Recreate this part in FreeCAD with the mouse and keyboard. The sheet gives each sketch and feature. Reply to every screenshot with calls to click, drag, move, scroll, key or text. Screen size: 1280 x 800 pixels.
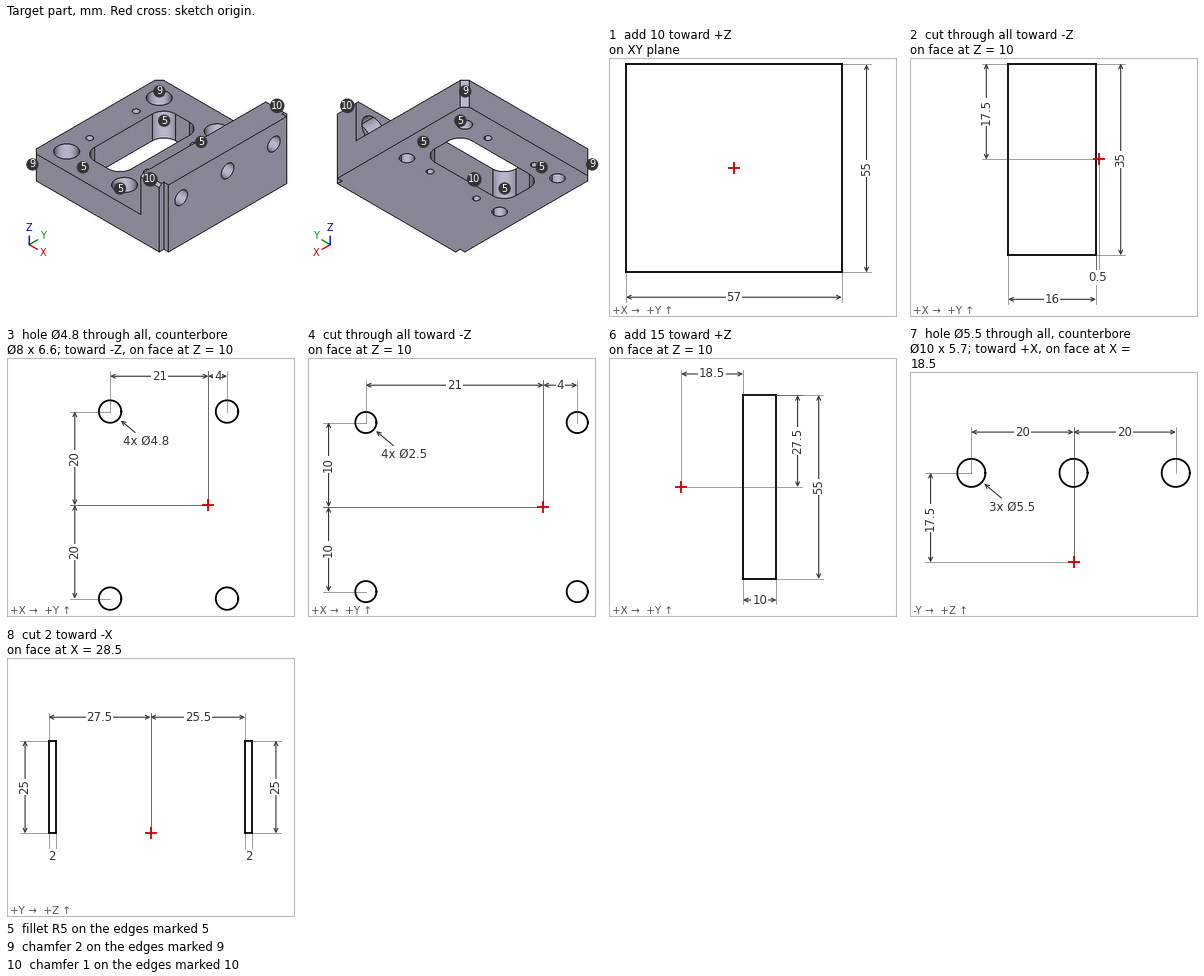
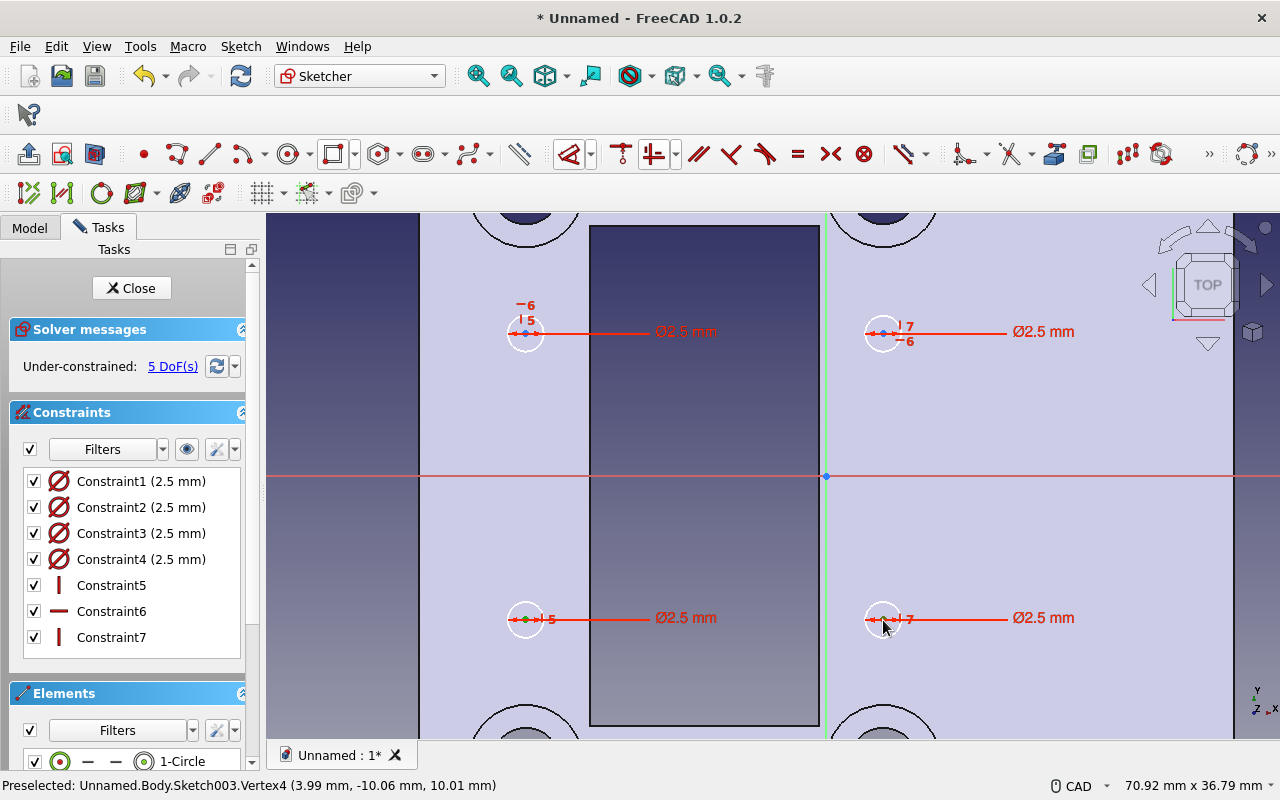
click(676, 154)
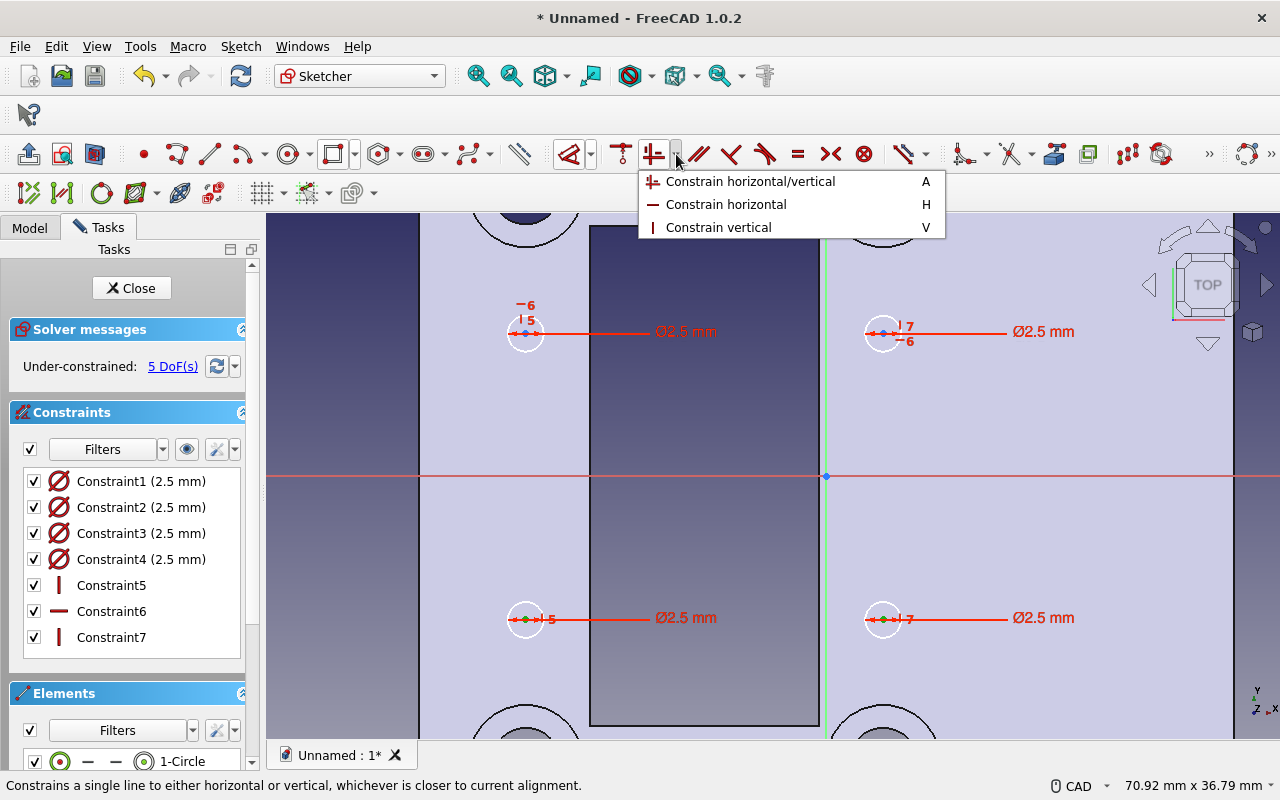
click(792, 204)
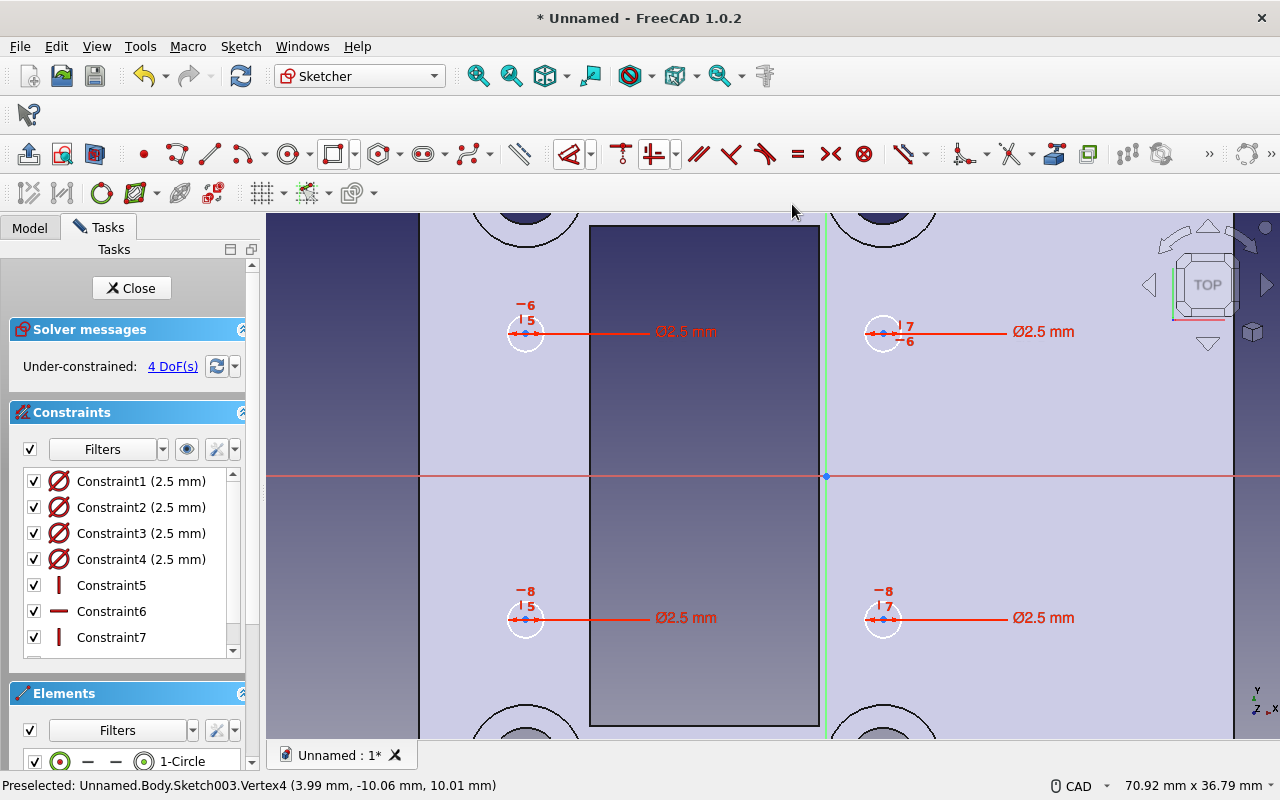
click(883, 334)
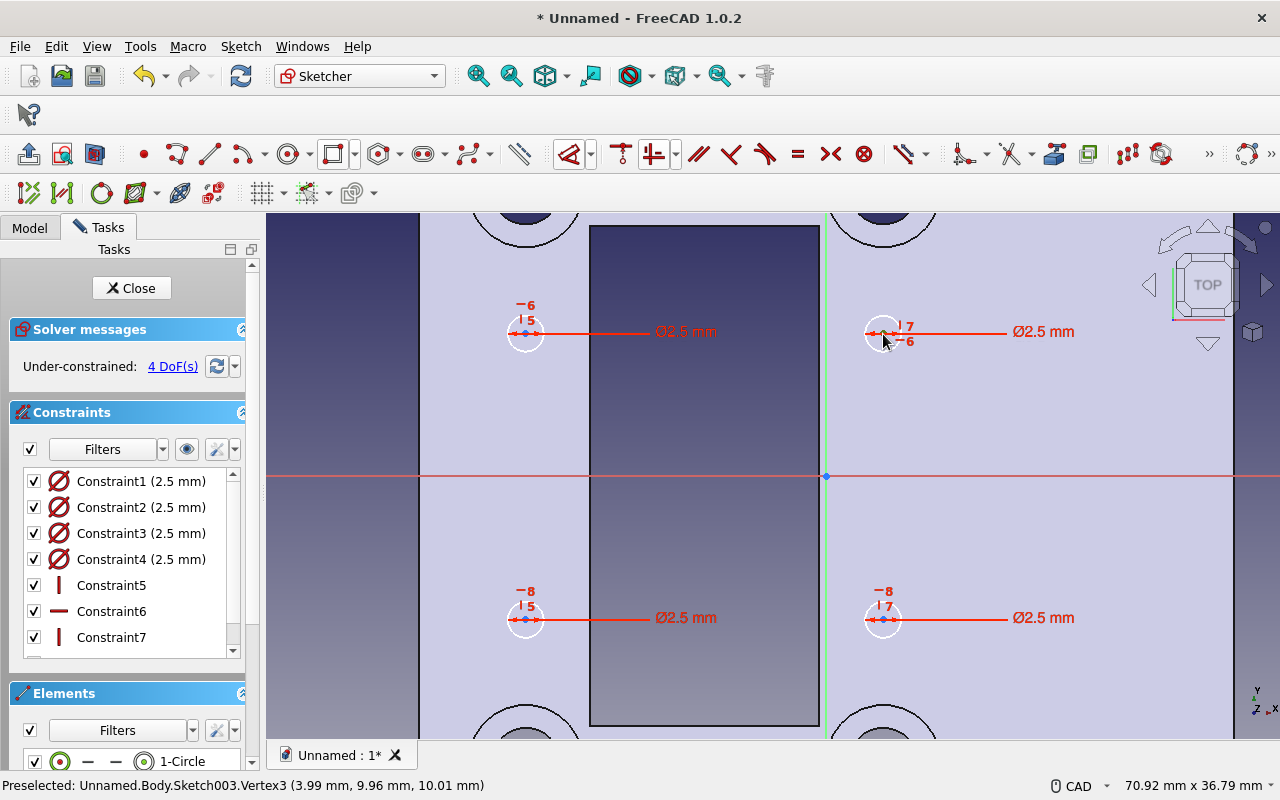
click(590, 154)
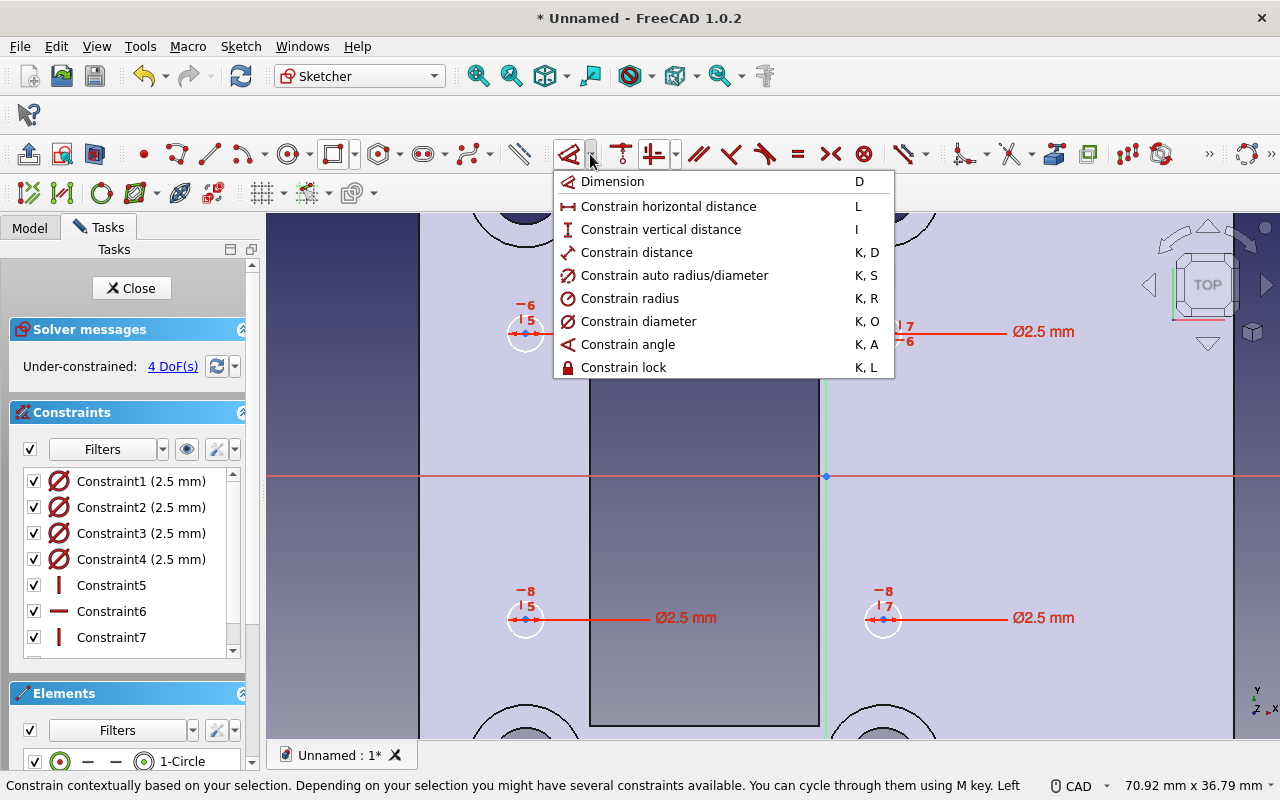
click(724, 206)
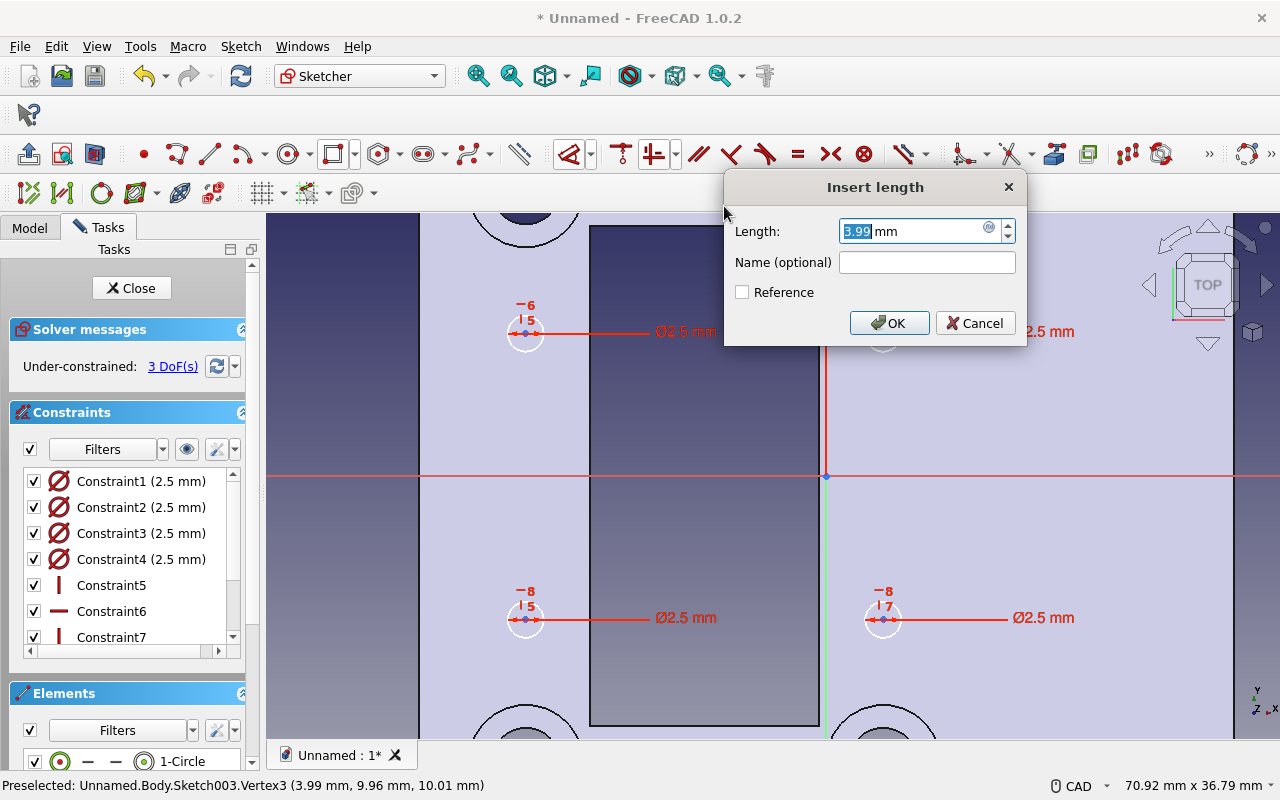
text(4)
key(Return)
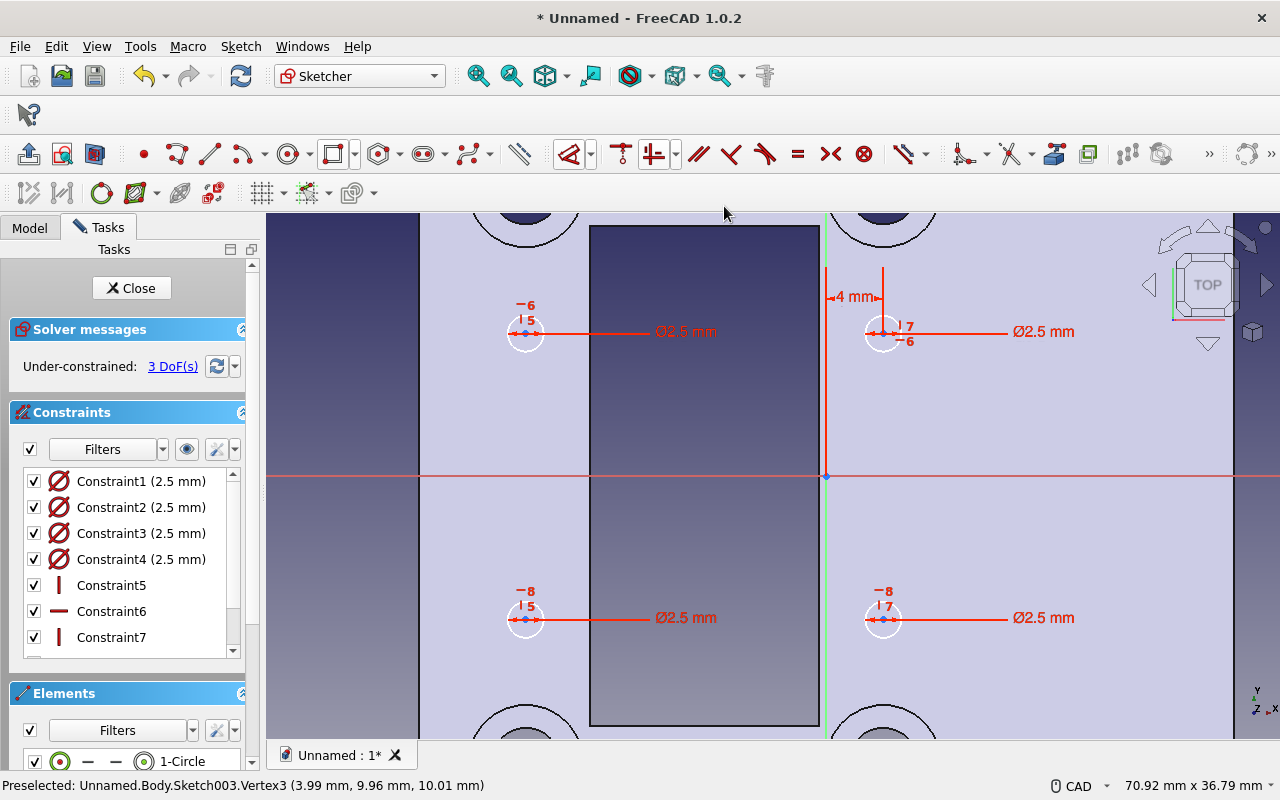
click(526, 334)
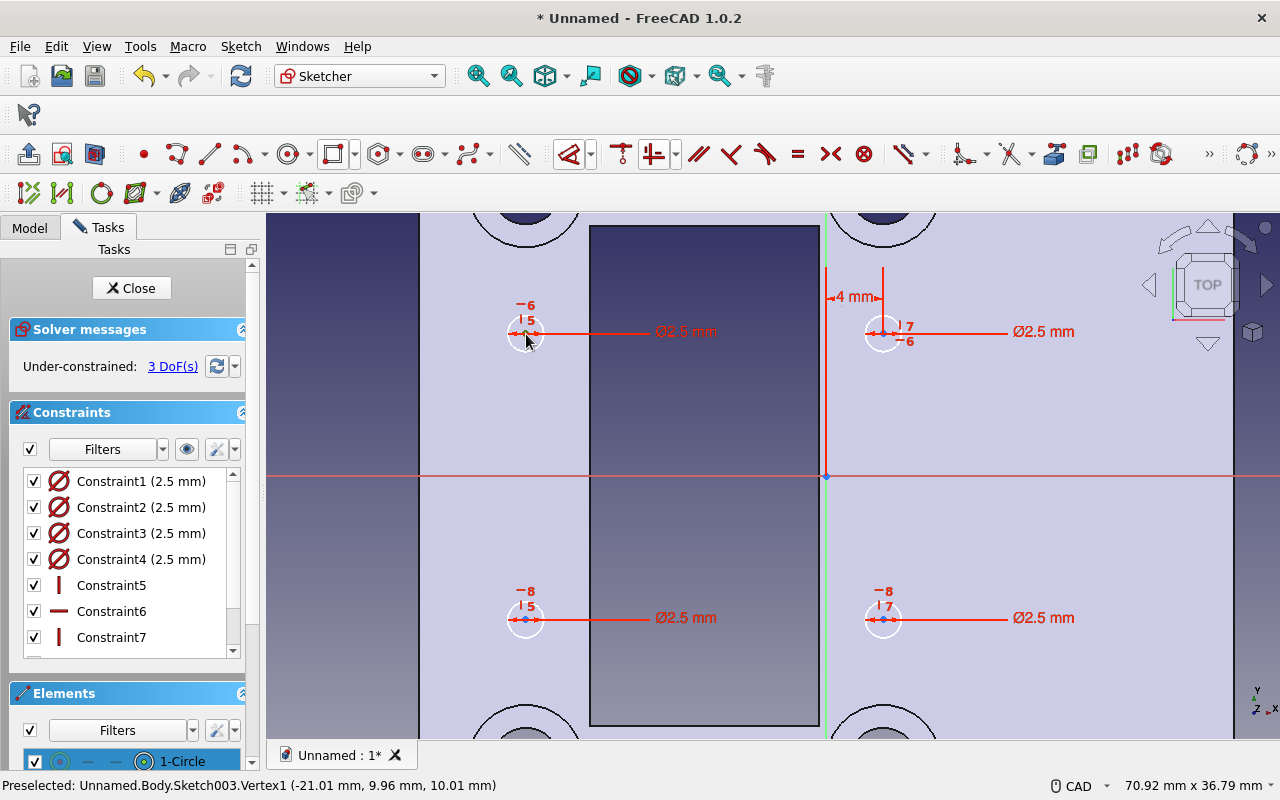
click(590, 154)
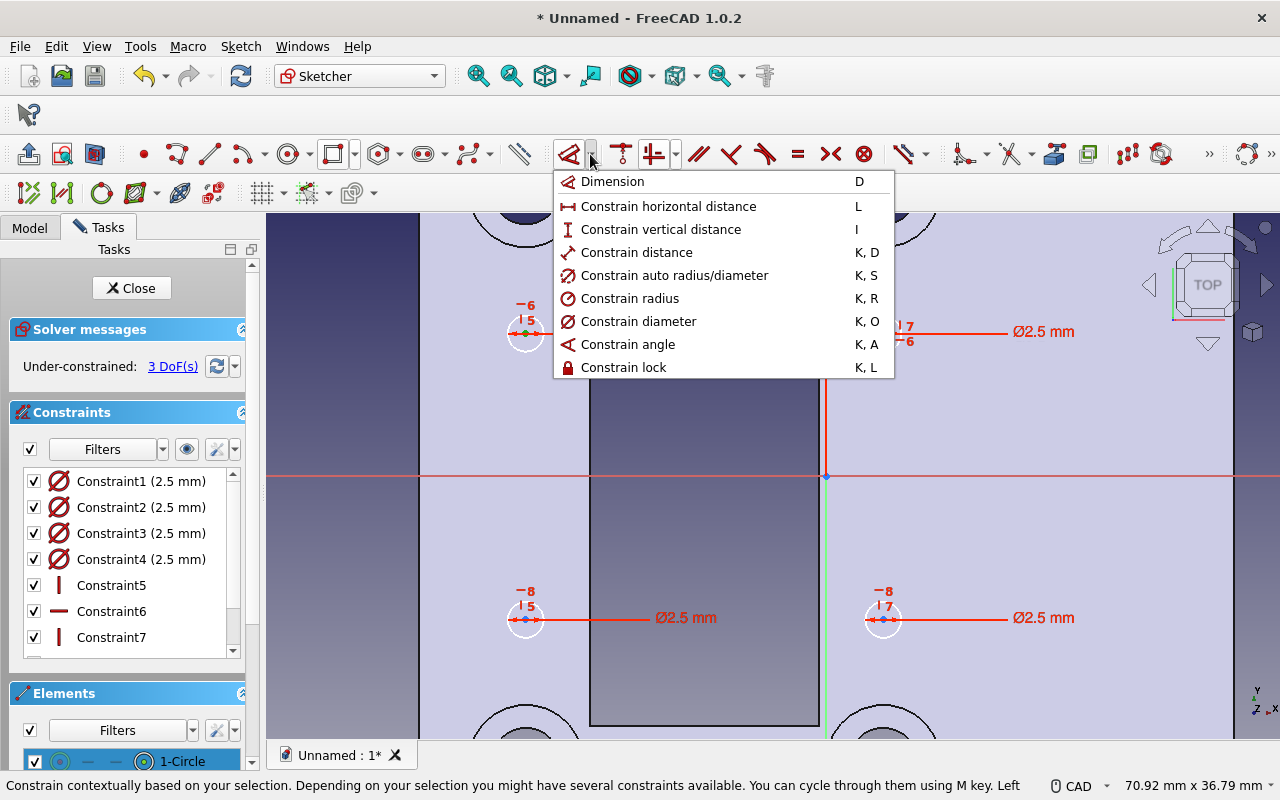
click(724, 206)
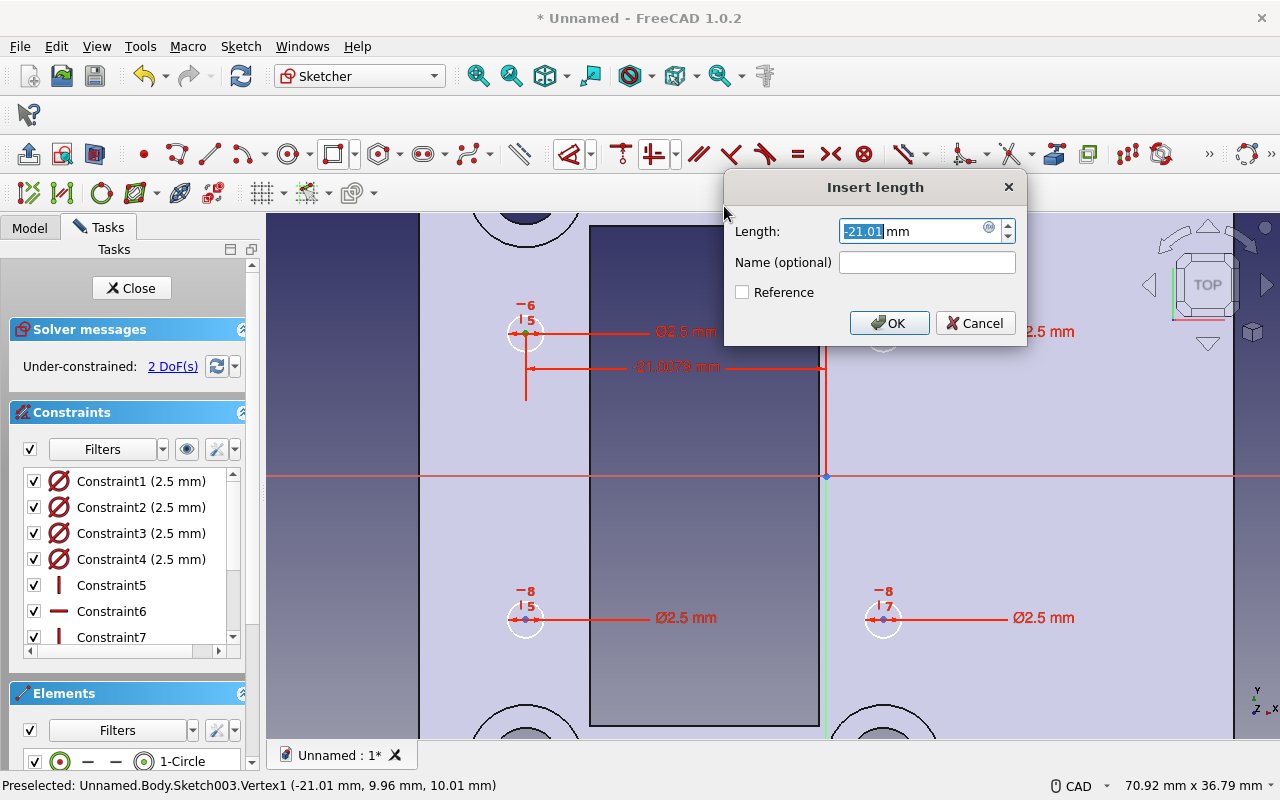
text(-21)
key(Return)